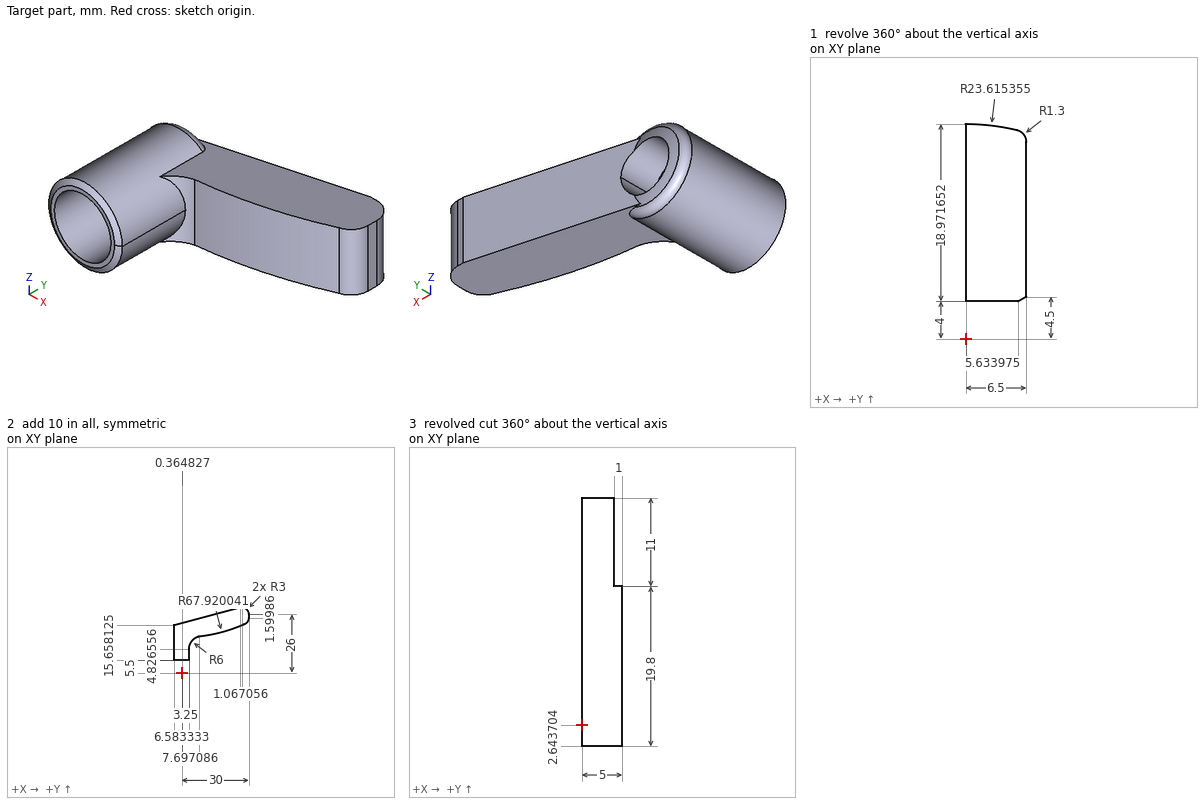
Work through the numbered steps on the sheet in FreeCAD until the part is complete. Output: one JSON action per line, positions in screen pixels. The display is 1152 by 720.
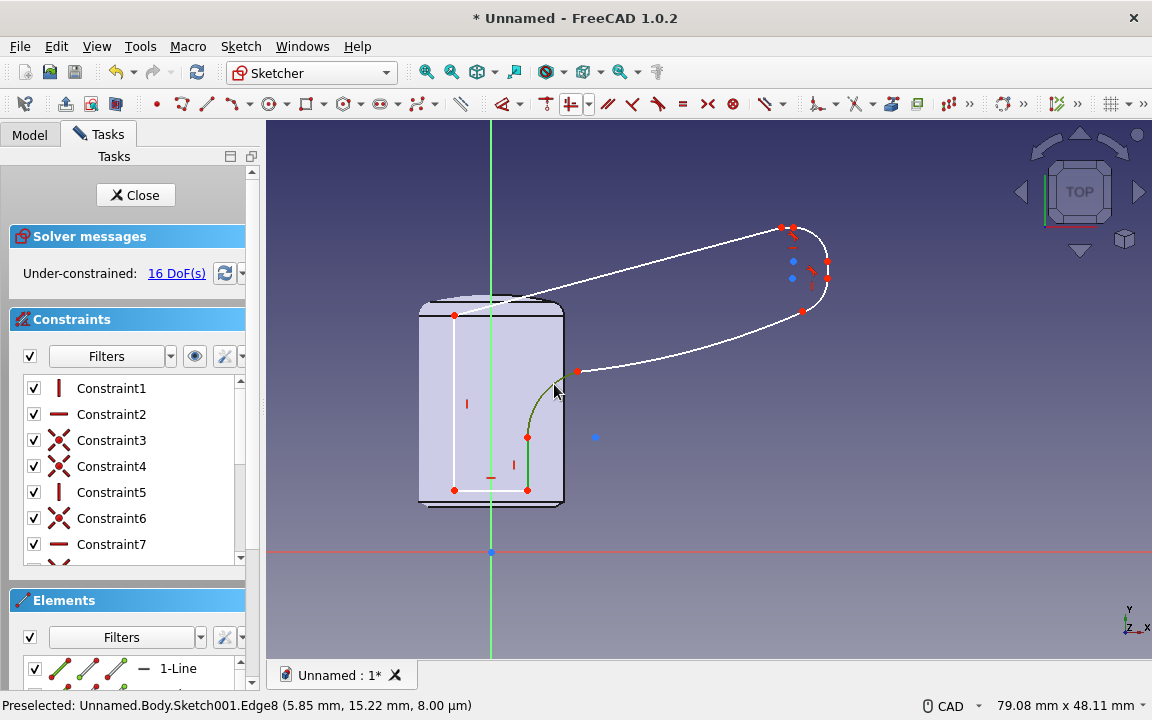
{"action": "key", "text": "t"}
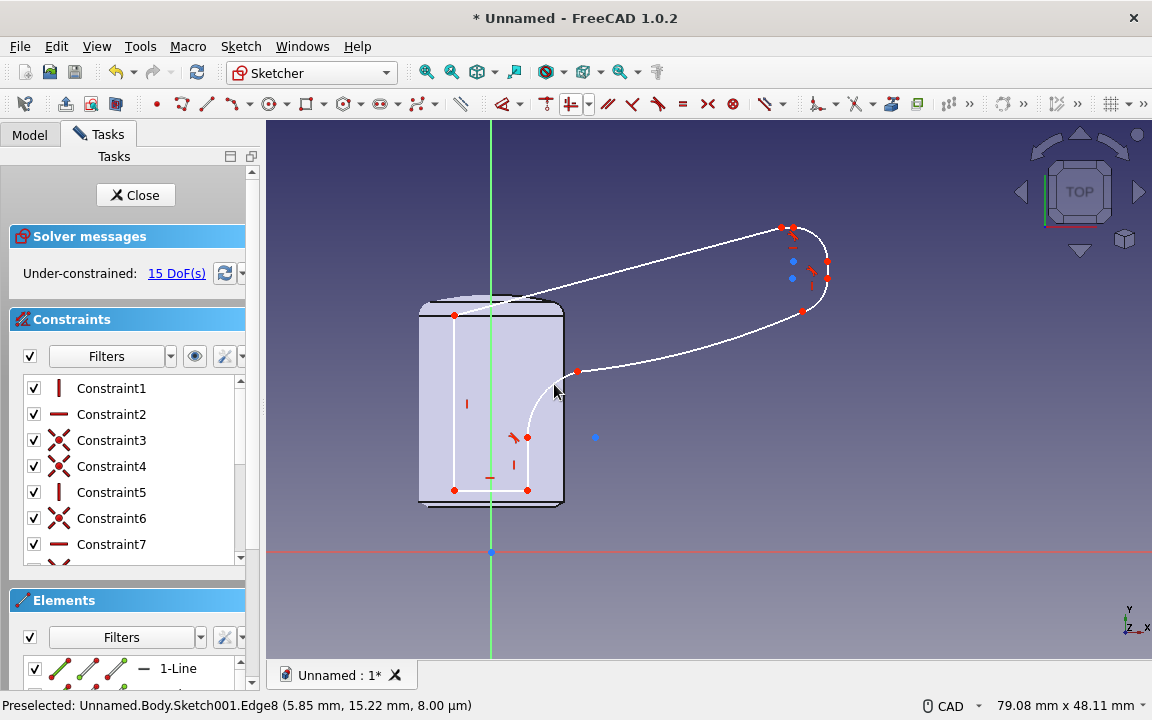
{"action": "left_click", "coordinate": [824, 246]}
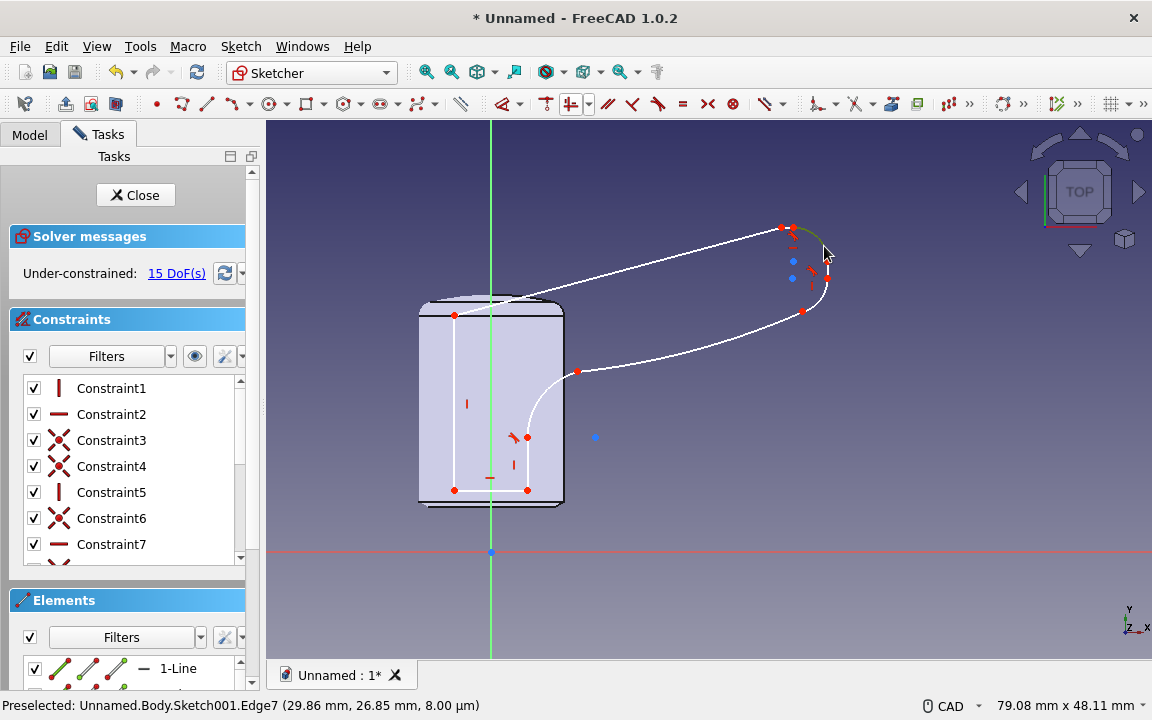
{"action": "left_click", "coordinate": [815, 306]}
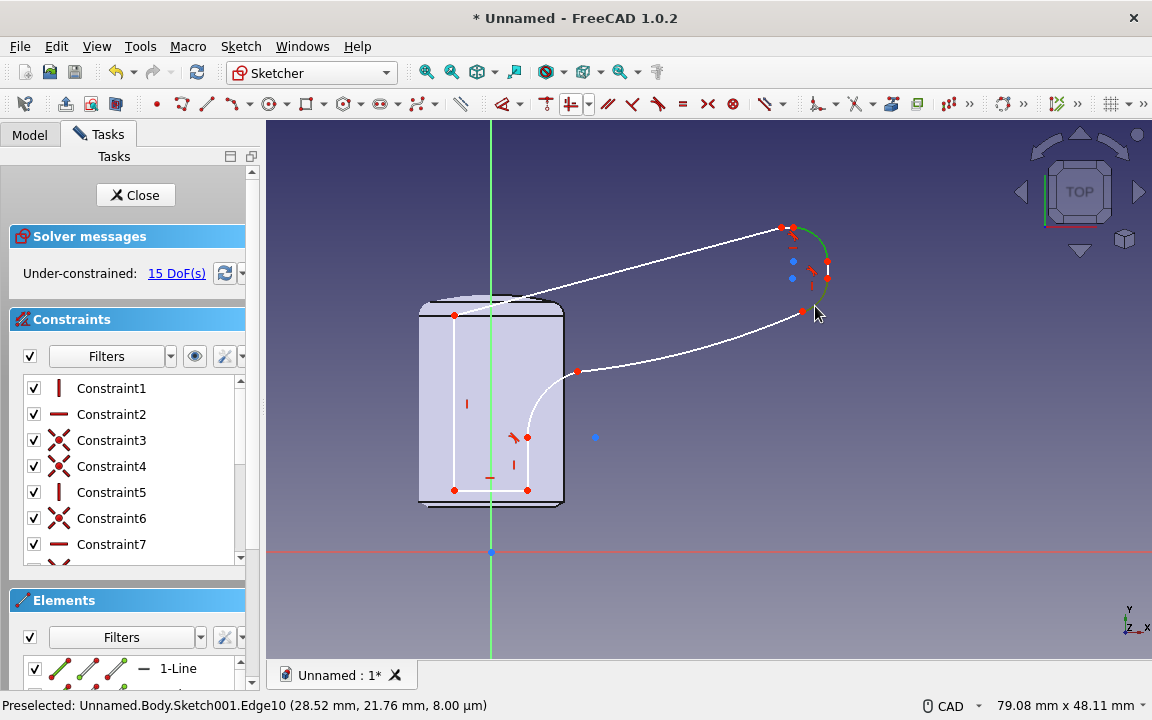
{"action": "key", "text": "e"}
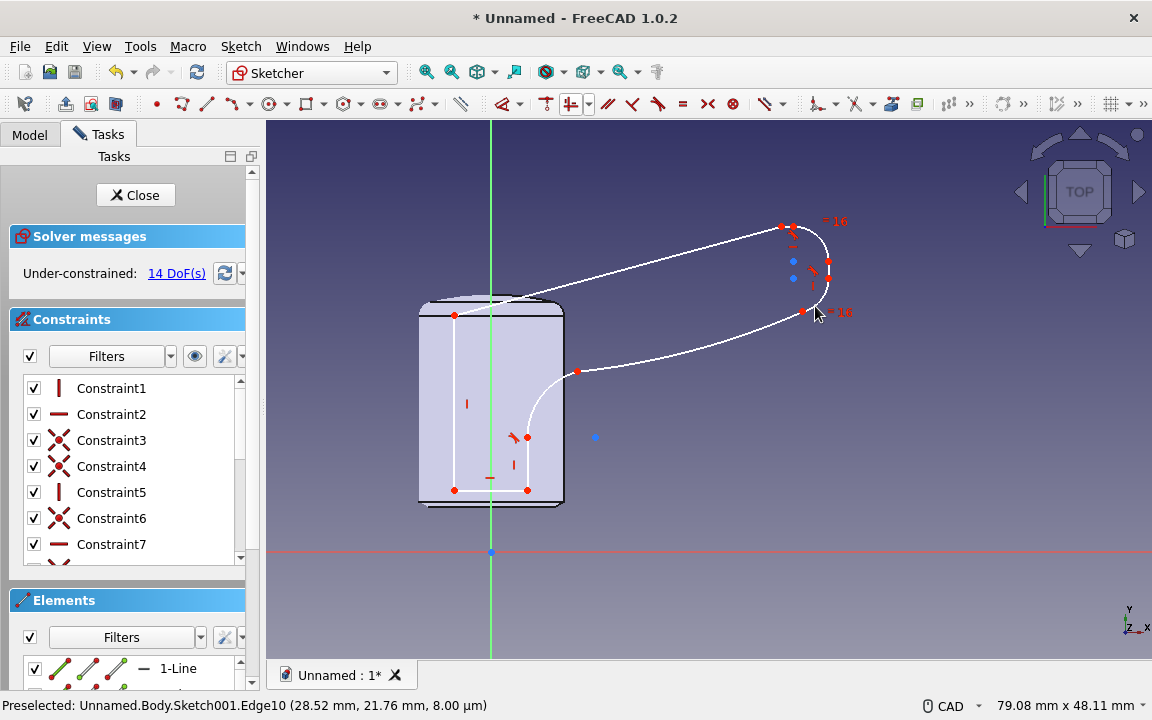
{"action": "key", "text": "d"}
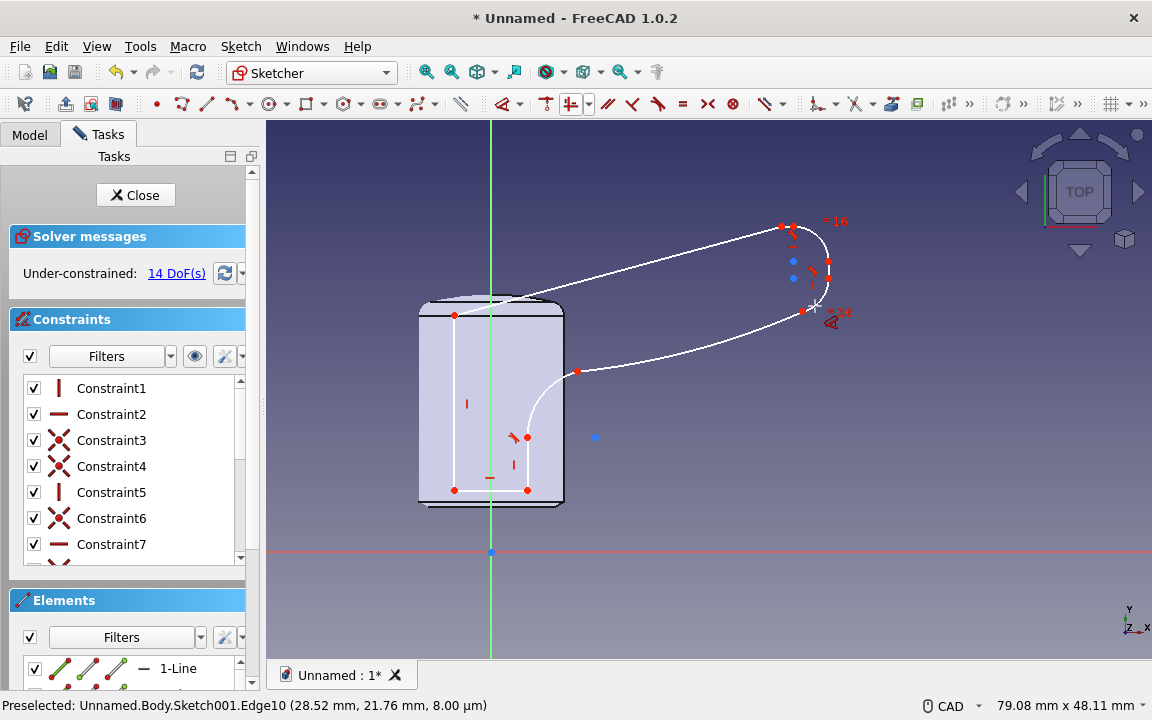
{"action": "left_click", "coordinate": [825, 246]}
{"action": "left_click", "coordinate": [854, 232]}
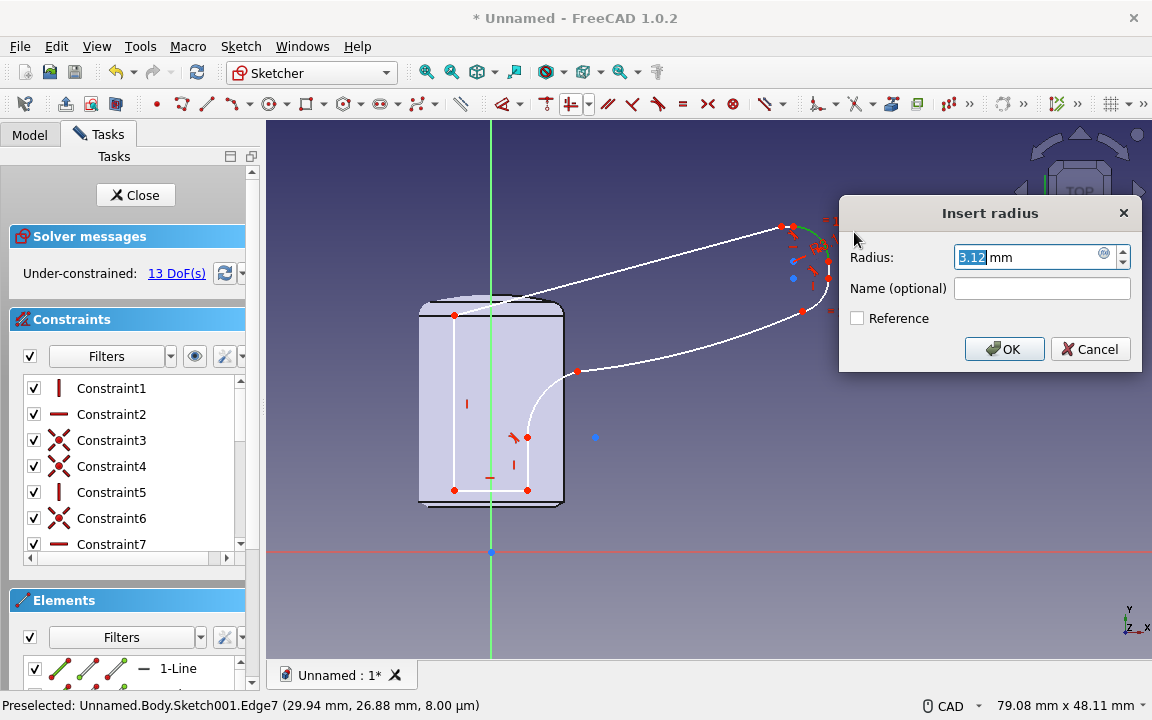
{"action": "type", "text": "3"}
{"action": "key", "text": "Return"}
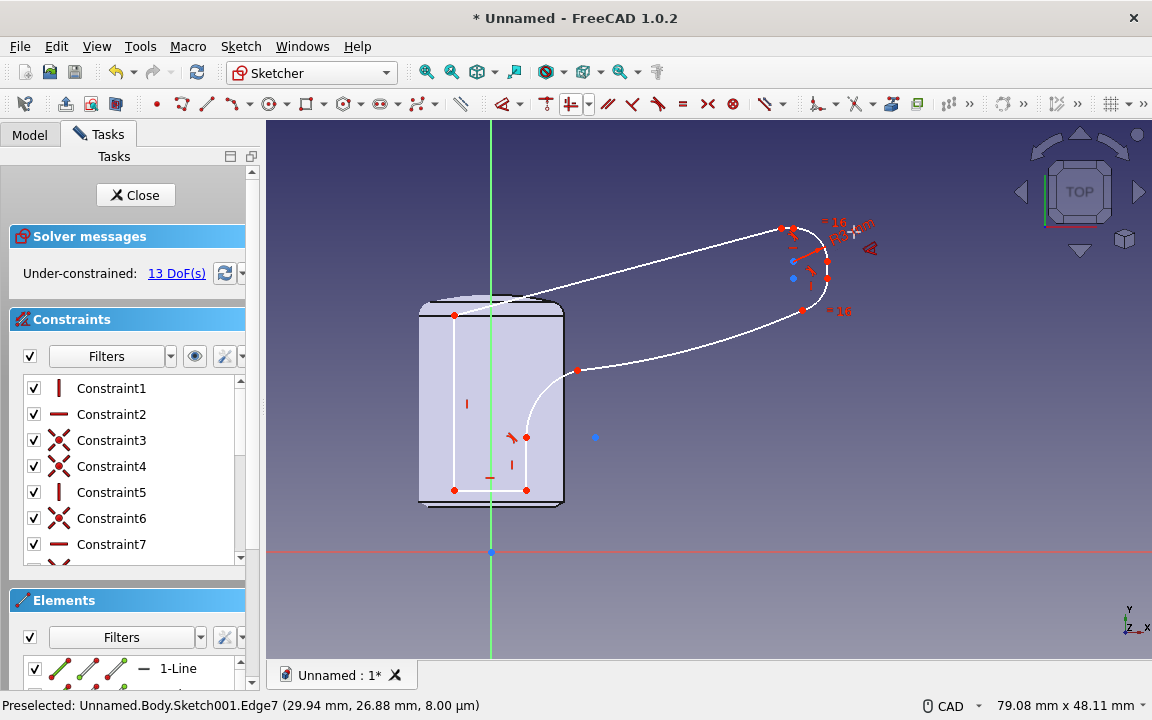
{"action": "left_click", "coordinate": [554, 382]}
{"action": "left_click", "coordinate": [535, 356]}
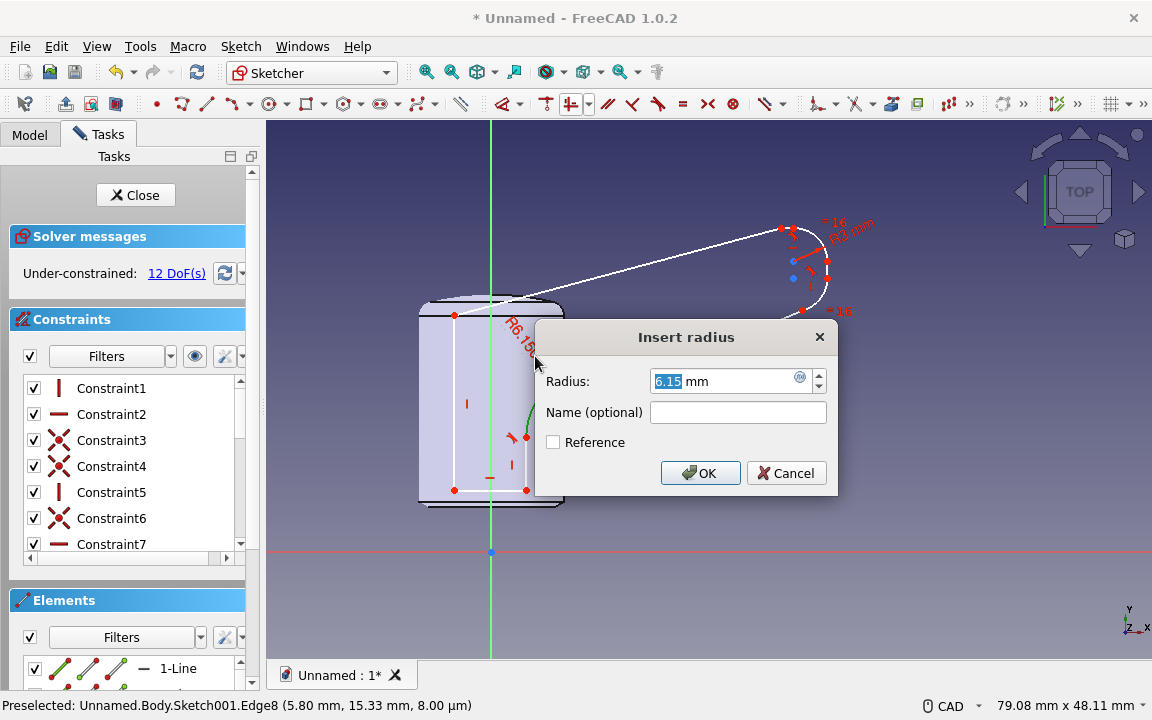
{"action": "type", "text": "6"}
{"action": "key", "text": "Return"}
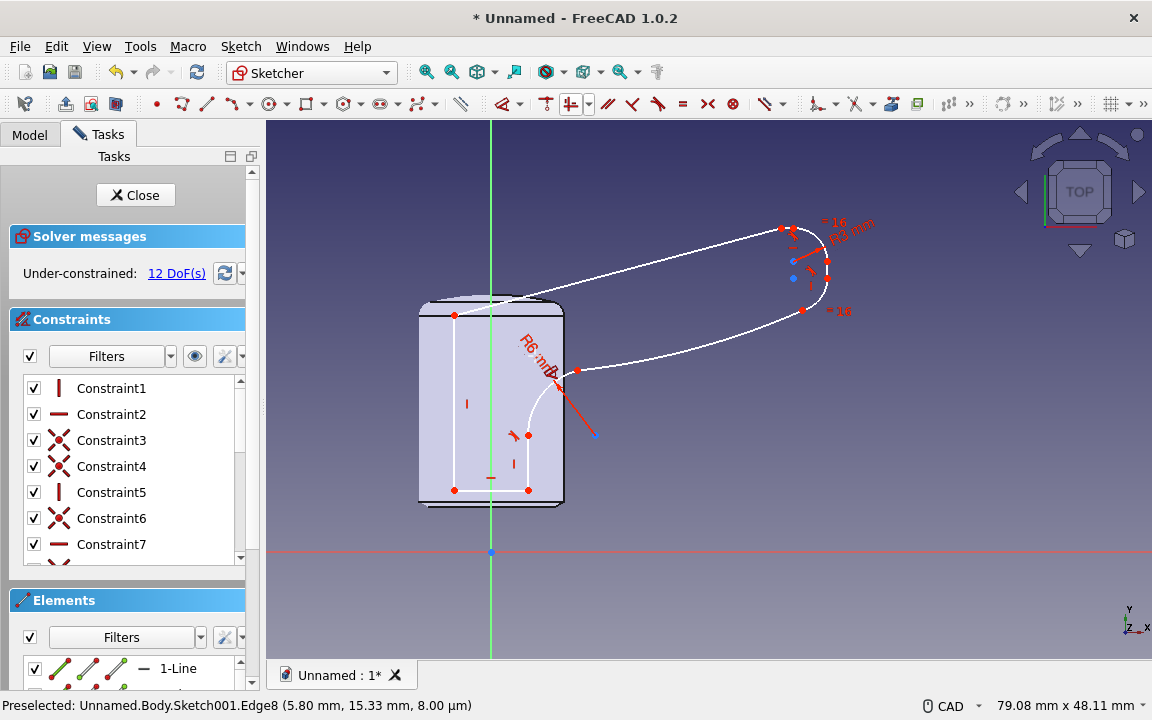
{"action": "left_click", "coordinate": [647, 360]}
{"action": "left_click", "coordinate": [653, 391]}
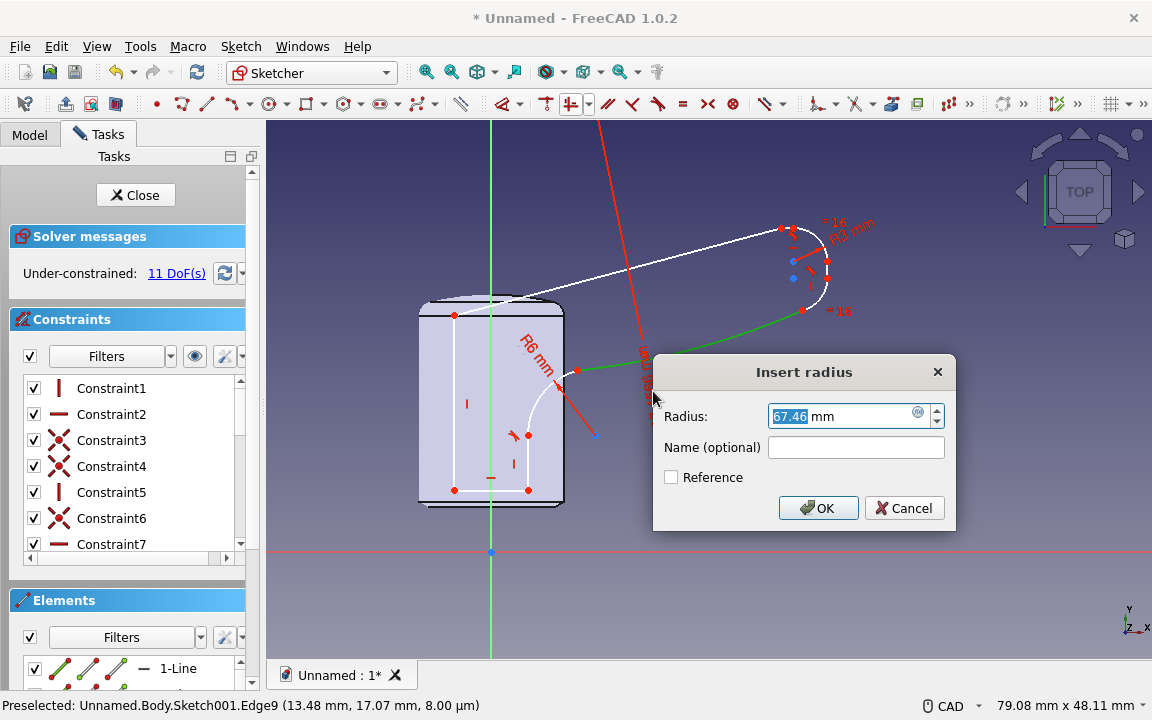
{"action": "type", "text": "67.920041"}
{"action": "key", "text": "Return"}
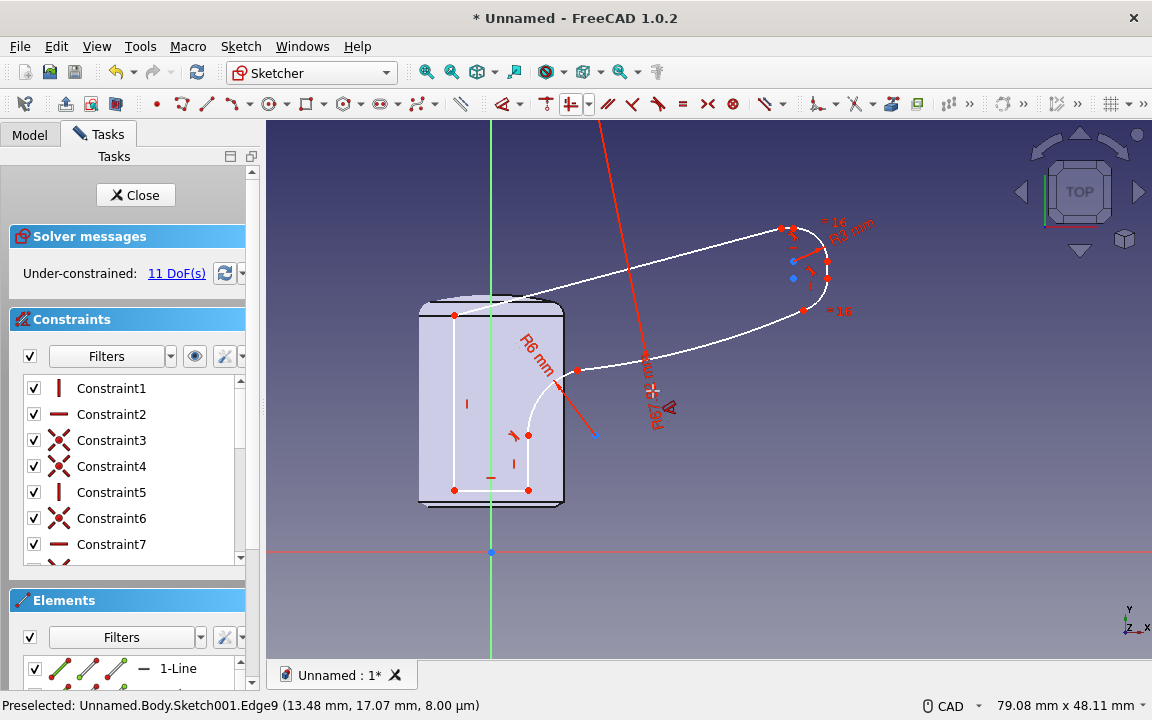
{"action": "left_click", "coordinate": [827, 278]}
{"action": "left_click", "coordinate": [659, 586]}